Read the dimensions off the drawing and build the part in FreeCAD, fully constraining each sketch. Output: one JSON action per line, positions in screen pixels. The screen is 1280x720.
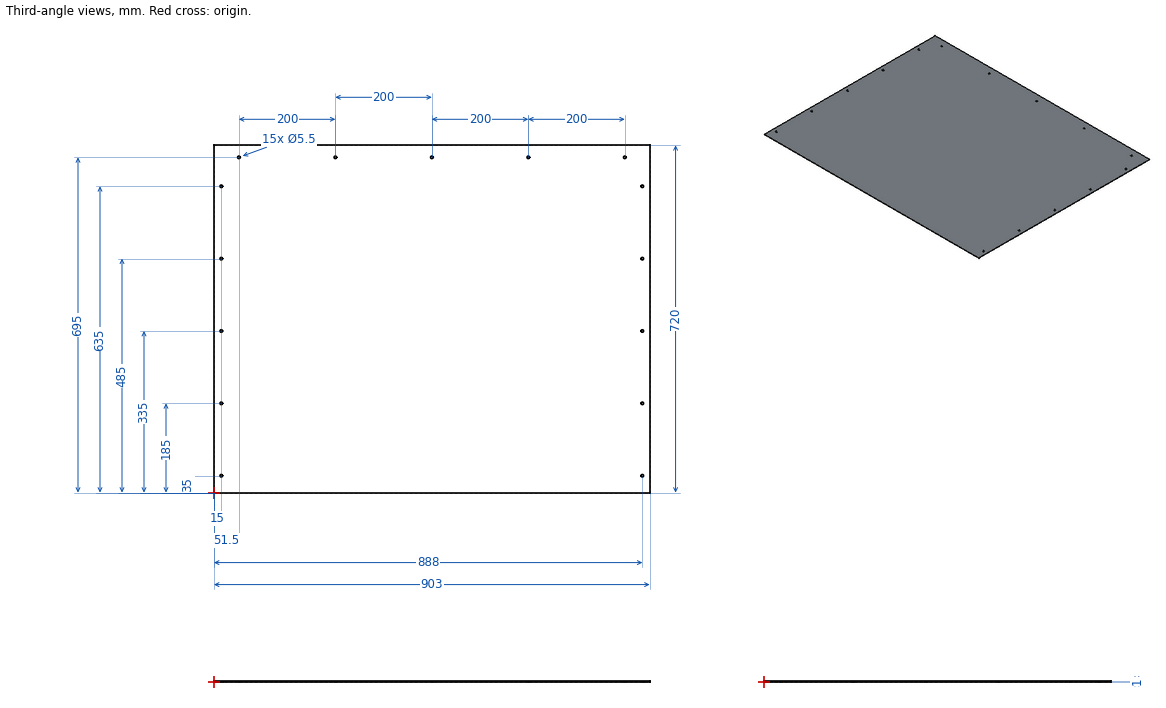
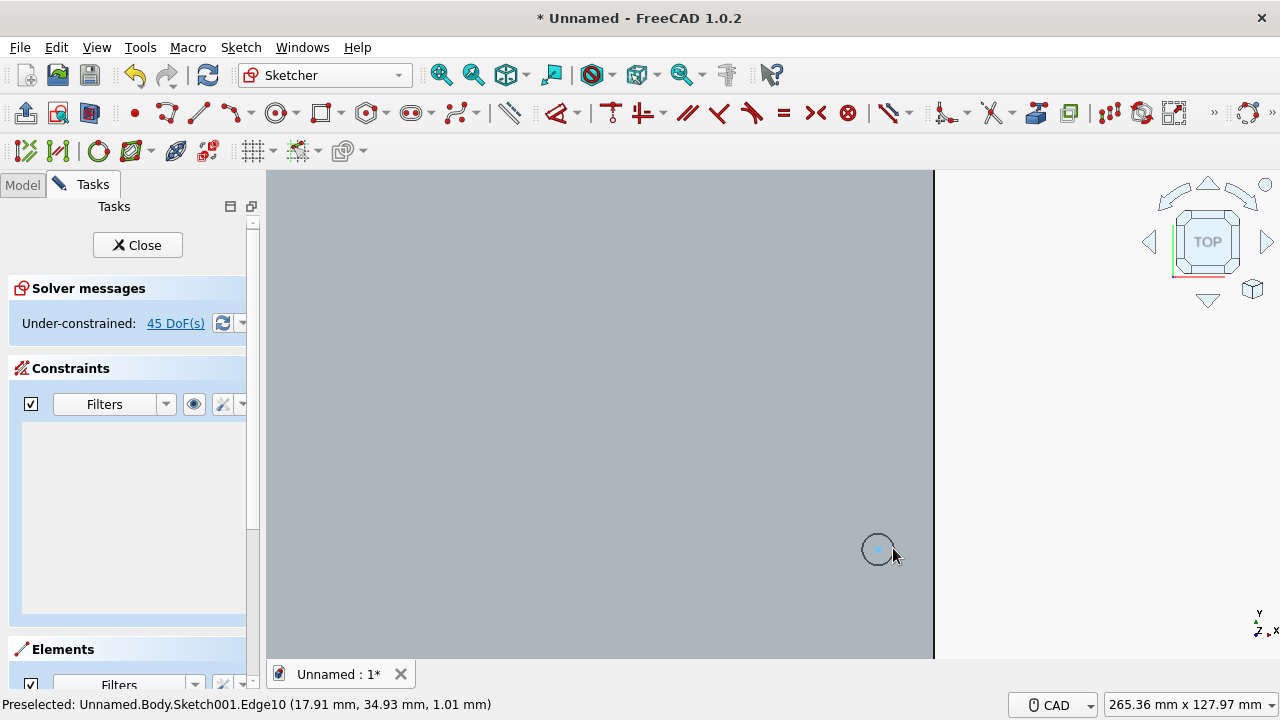
{"action": "left_click", "coordinate": [889, 538]}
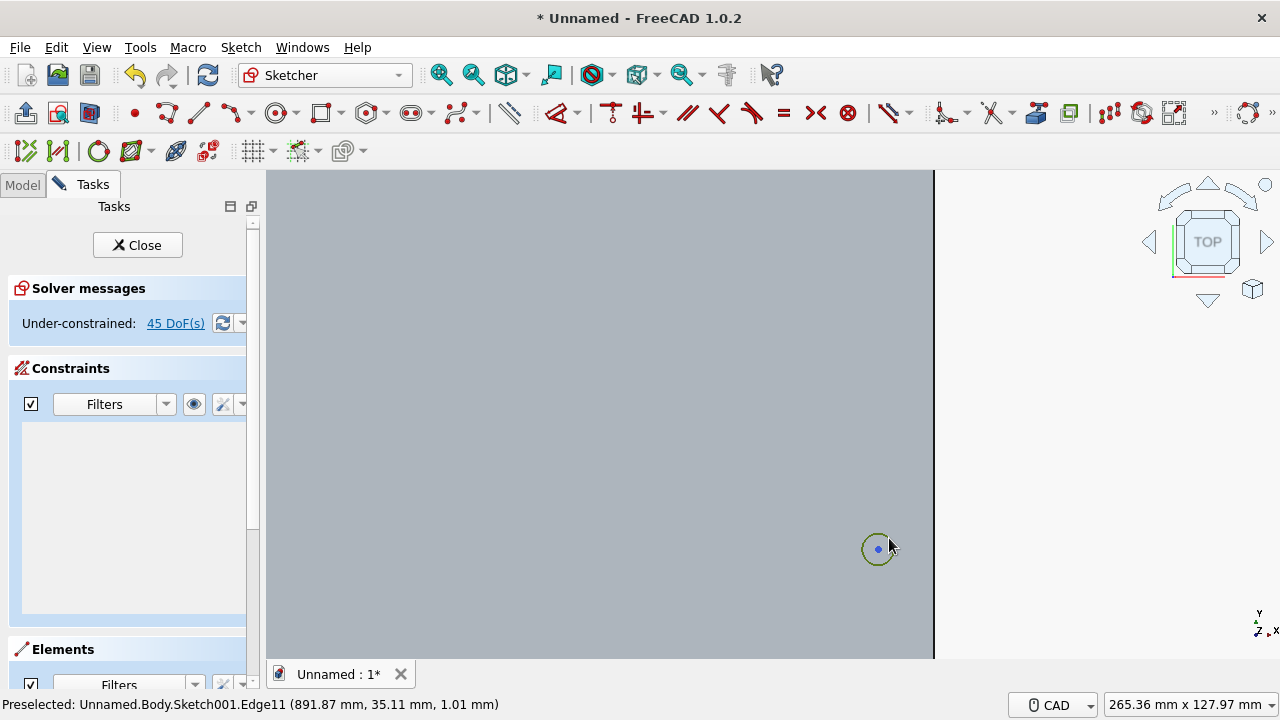
{"action": "scroll", "coordinate": [894, 548], "scroll_direction": "down", "scroll_amount": 11}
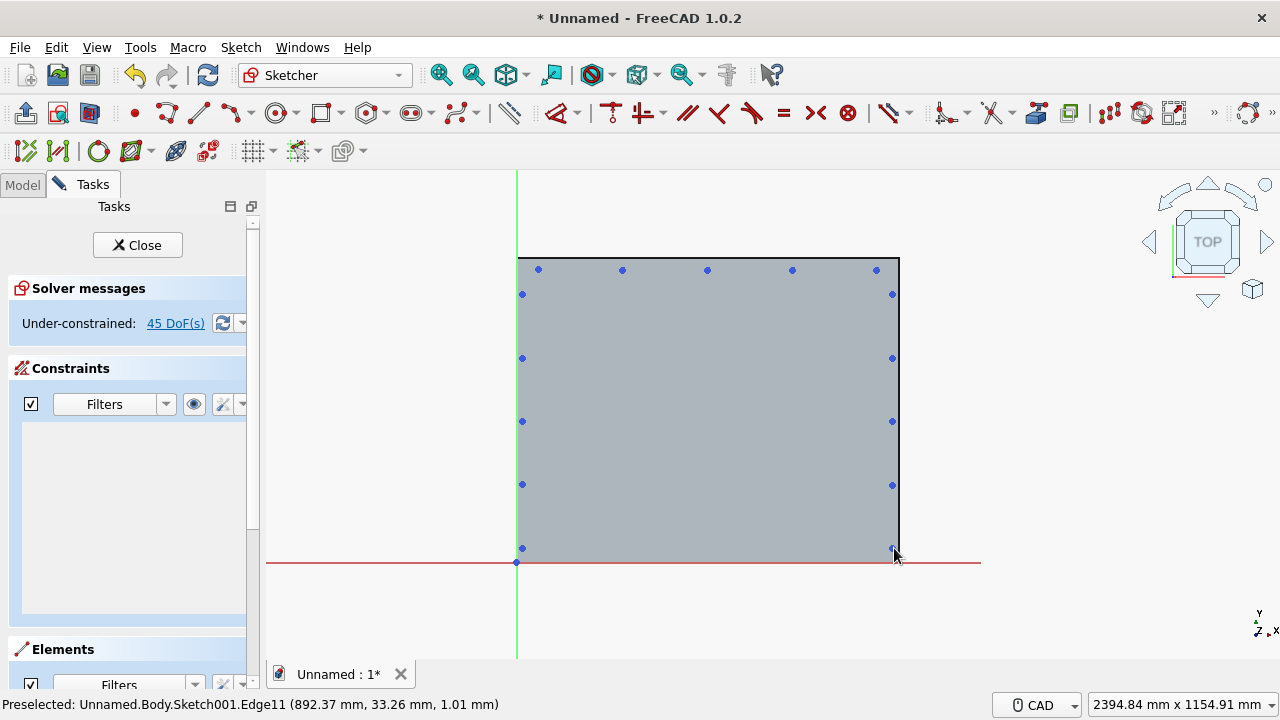
{"action": "scroll", "coordinate": [894, 484], "scroll_direction": "up", "scroll_amount": 10}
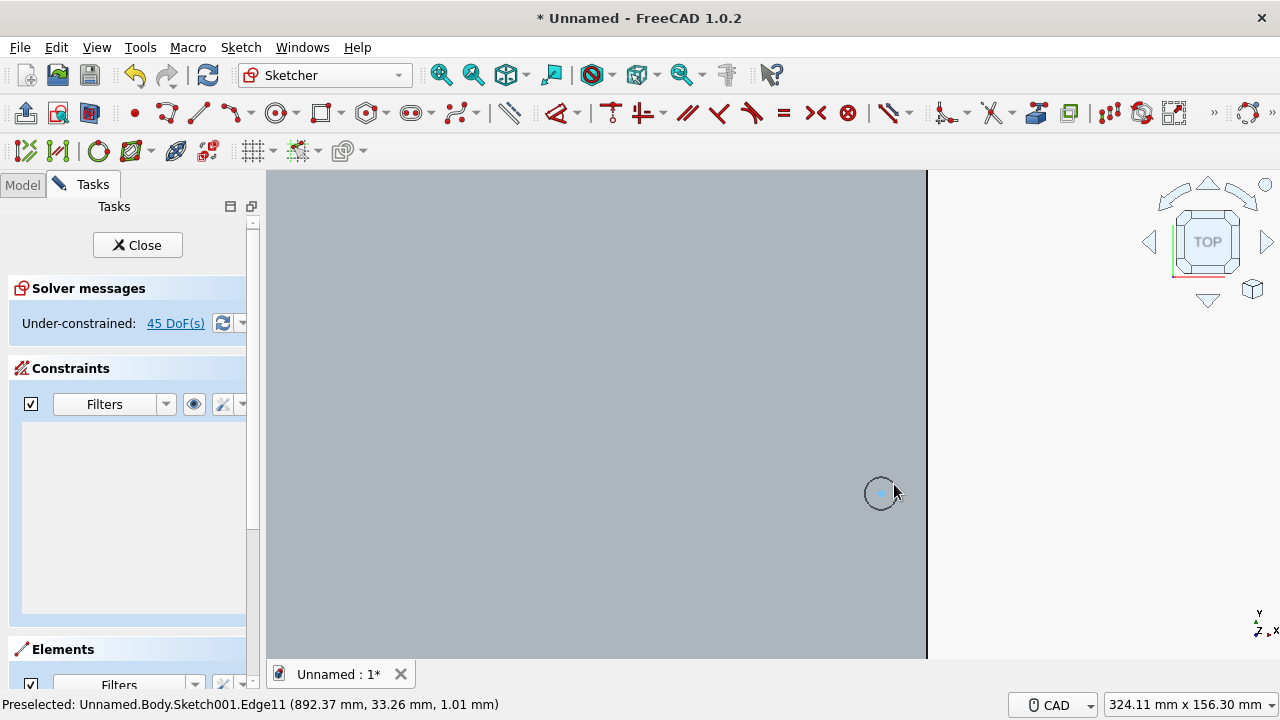
{"action": "left_click", "coordinate": [892, 482]}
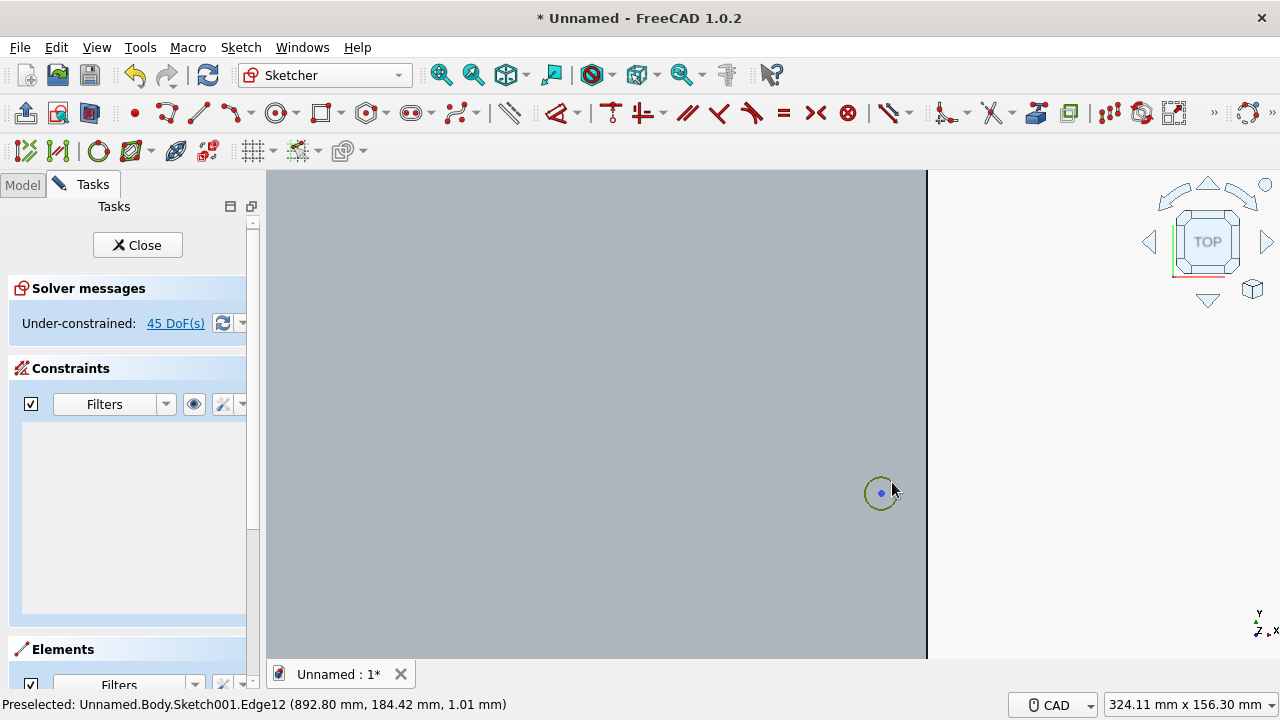
{"action": "scroll", "coordinate": [894, 484], "scroll_direction": "down", "scroll_amount": 10}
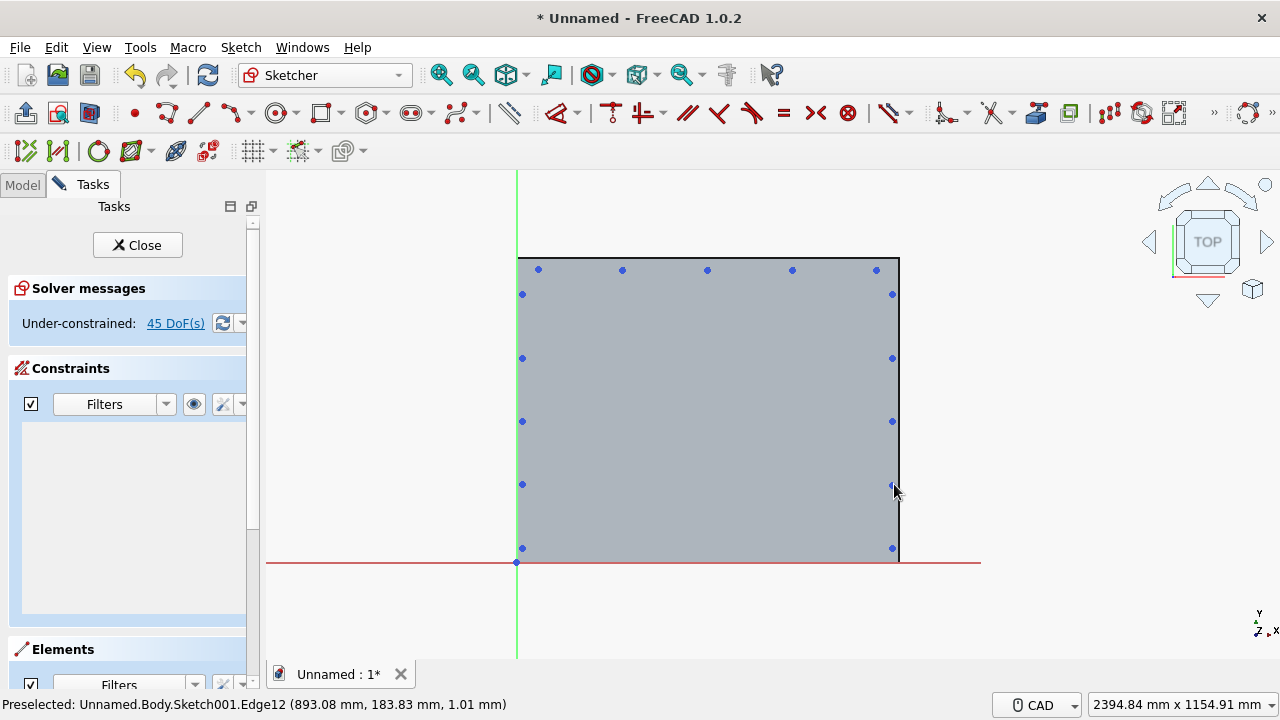
{"action": "scroll", "coordinate": [894, 421], "scroll_direction": "up", "scroll_amount": 11}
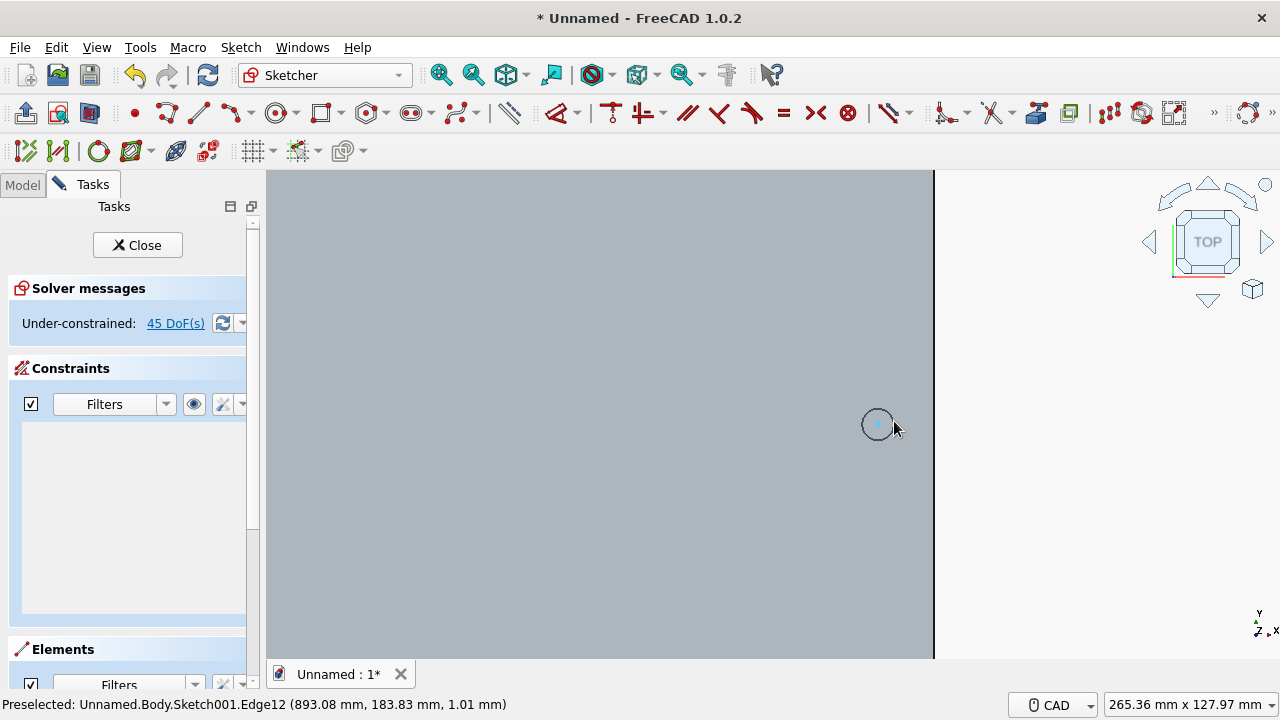
{"action": "left_click", "coordinate": [889, 413]}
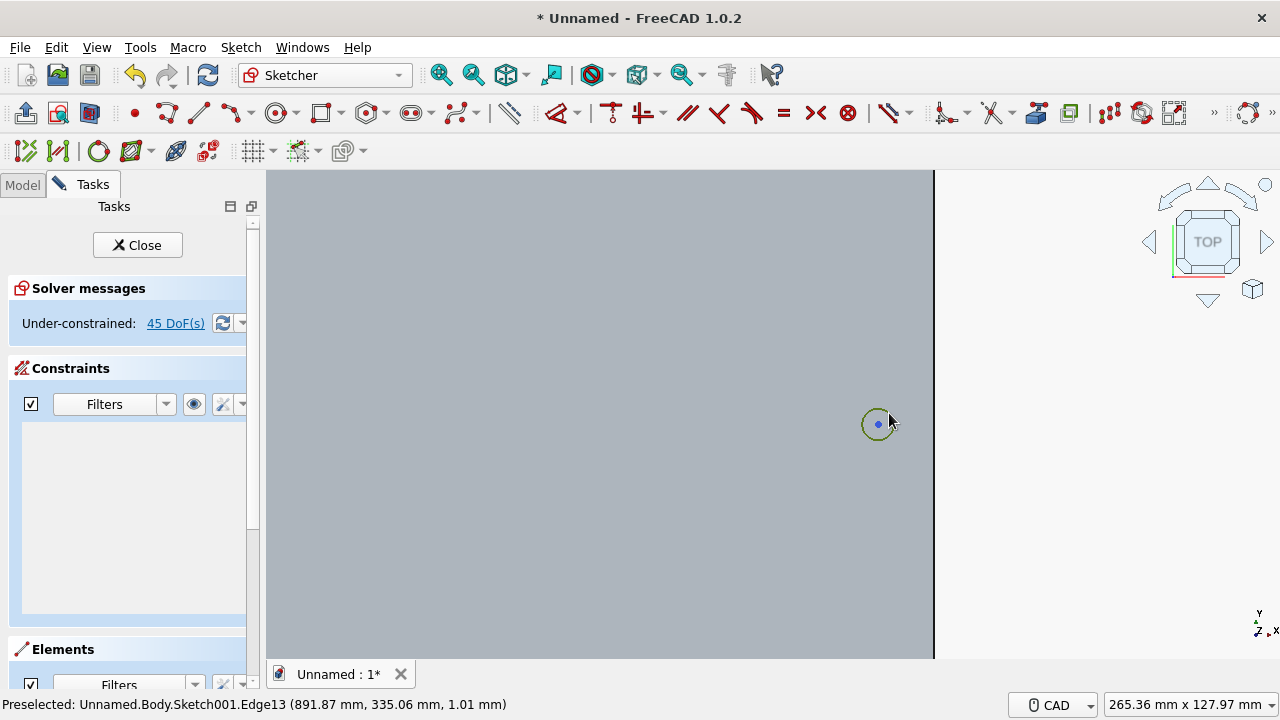
{"action": "scroll", "coordinate": [894, 421], "scroll_direction": "down", "scroll_amount": 11}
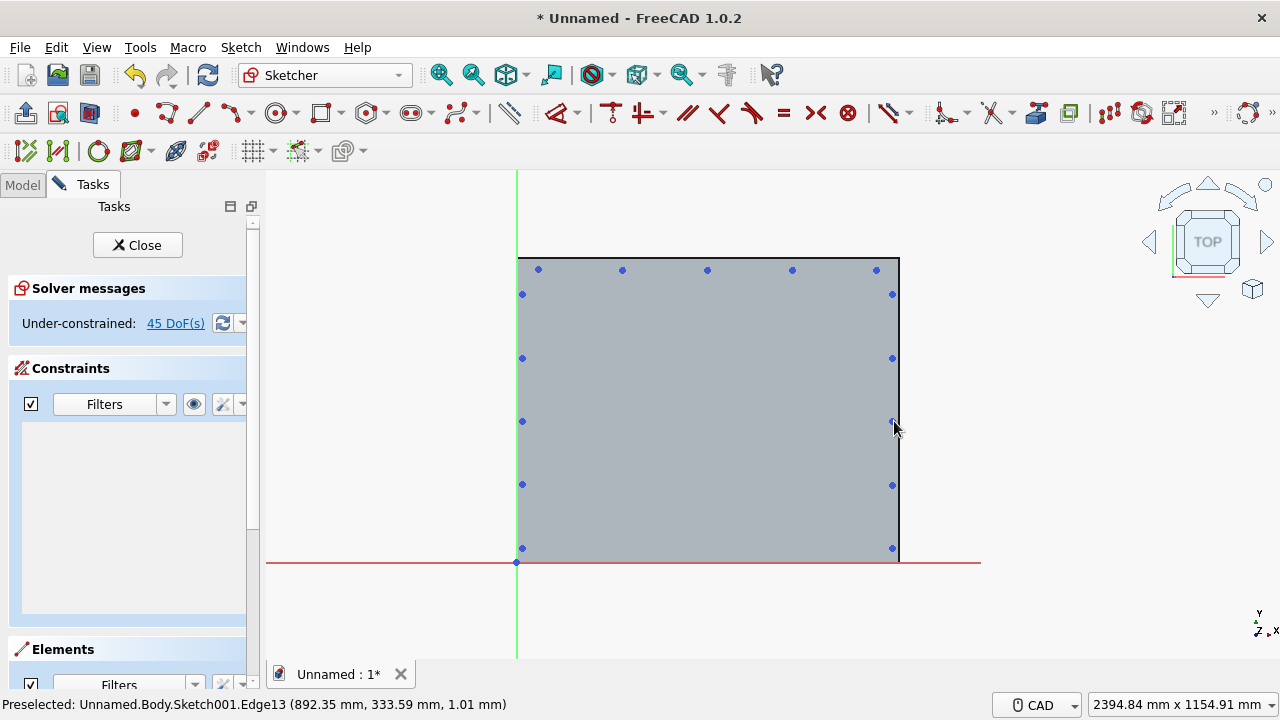
{"action": "scroll", "coordinate": [894, 357], "scroll_direction": "up", "scroll_amount": 10}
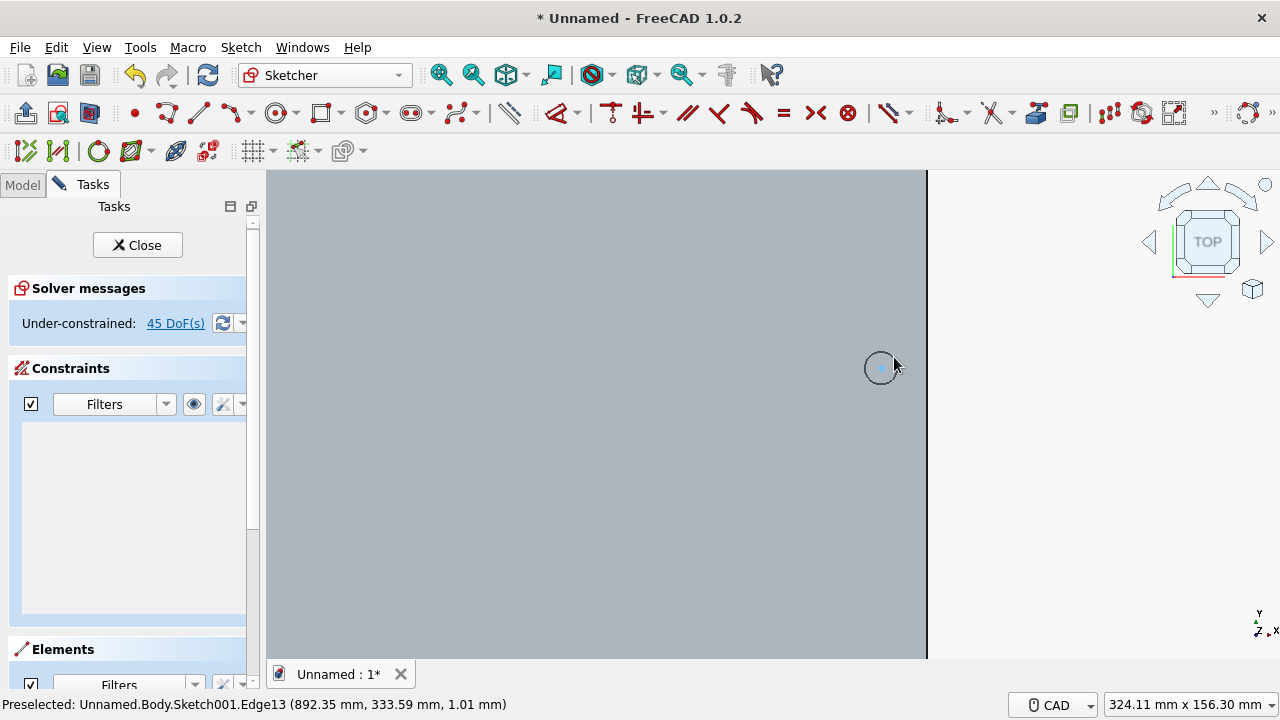
{"action": "left_click", "coordinate": [892, 357]}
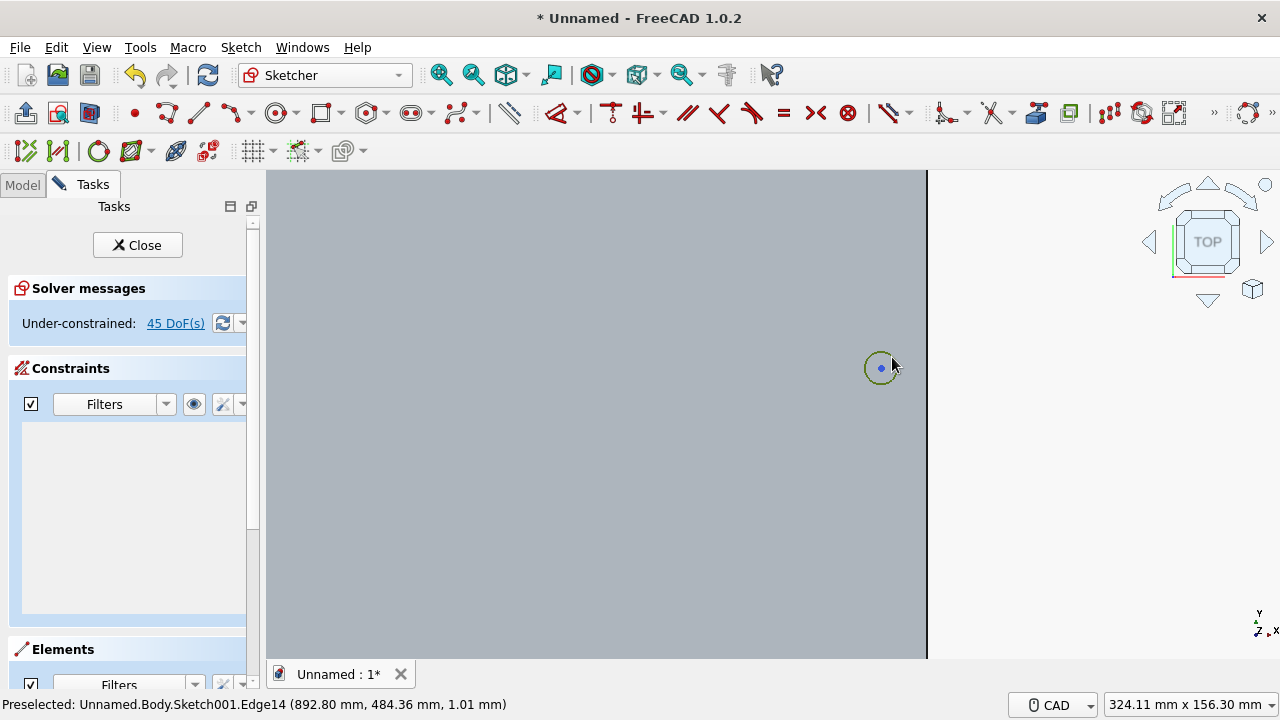
{"action": "scroll", "coordinate": [894, 357], "scroll_direction": "down", "scroll_amount": 10}